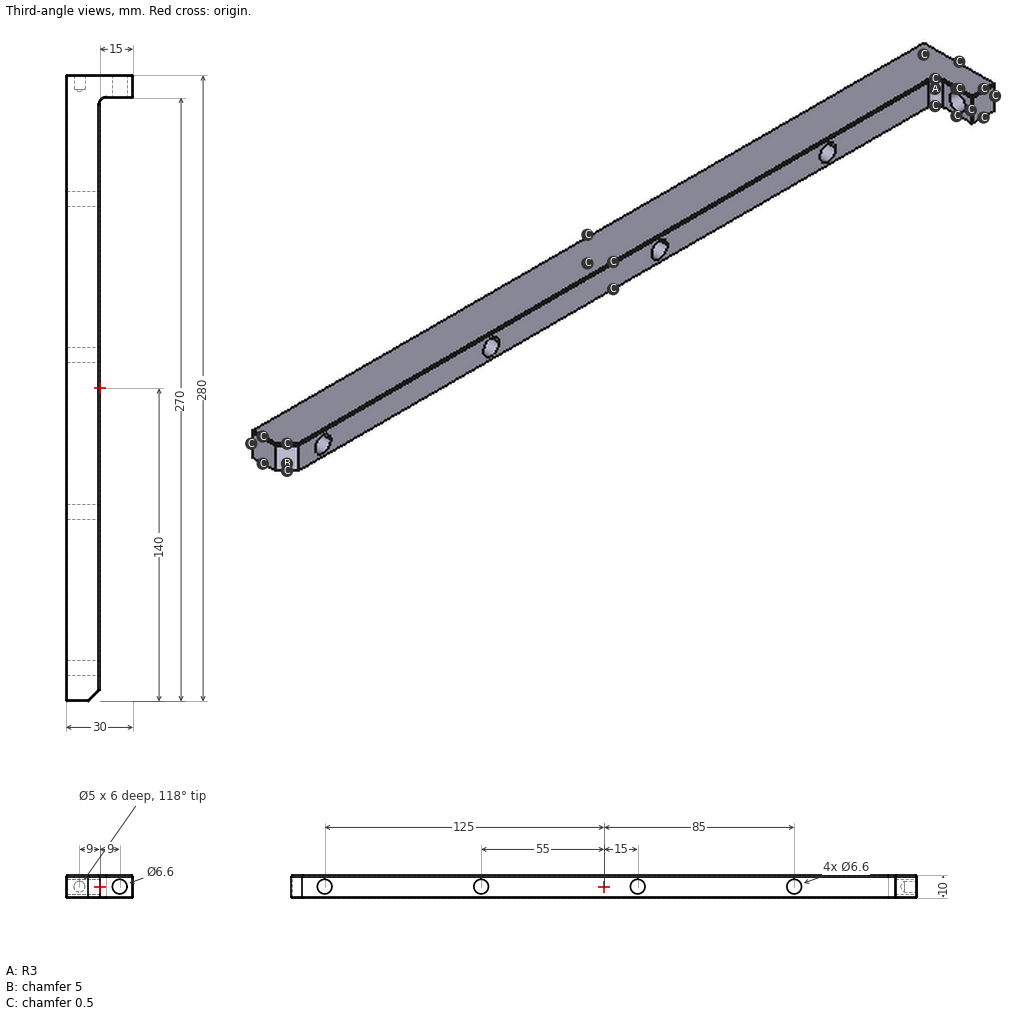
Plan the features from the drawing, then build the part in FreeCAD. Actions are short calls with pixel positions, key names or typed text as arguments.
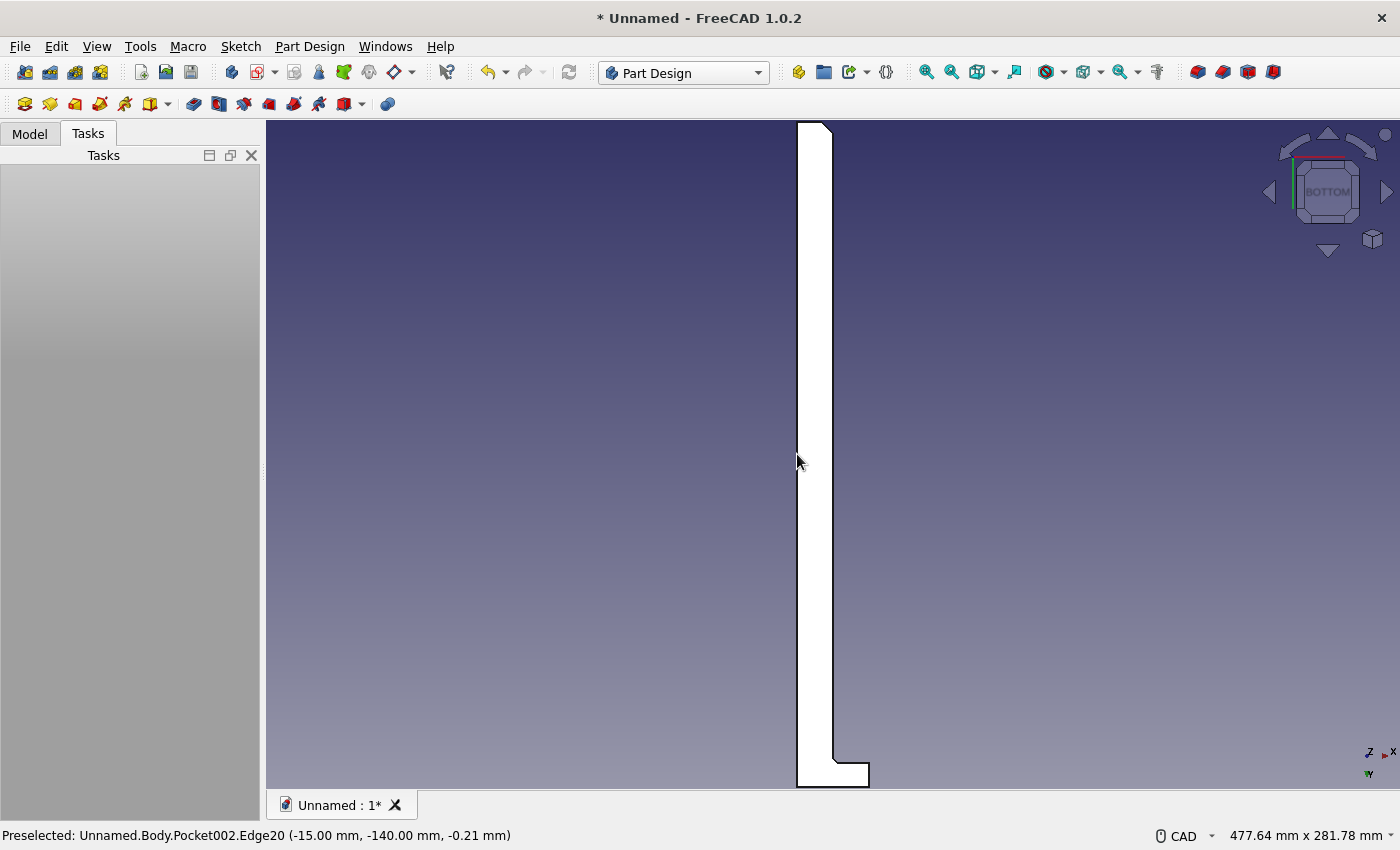
click(813, 738, ctrl)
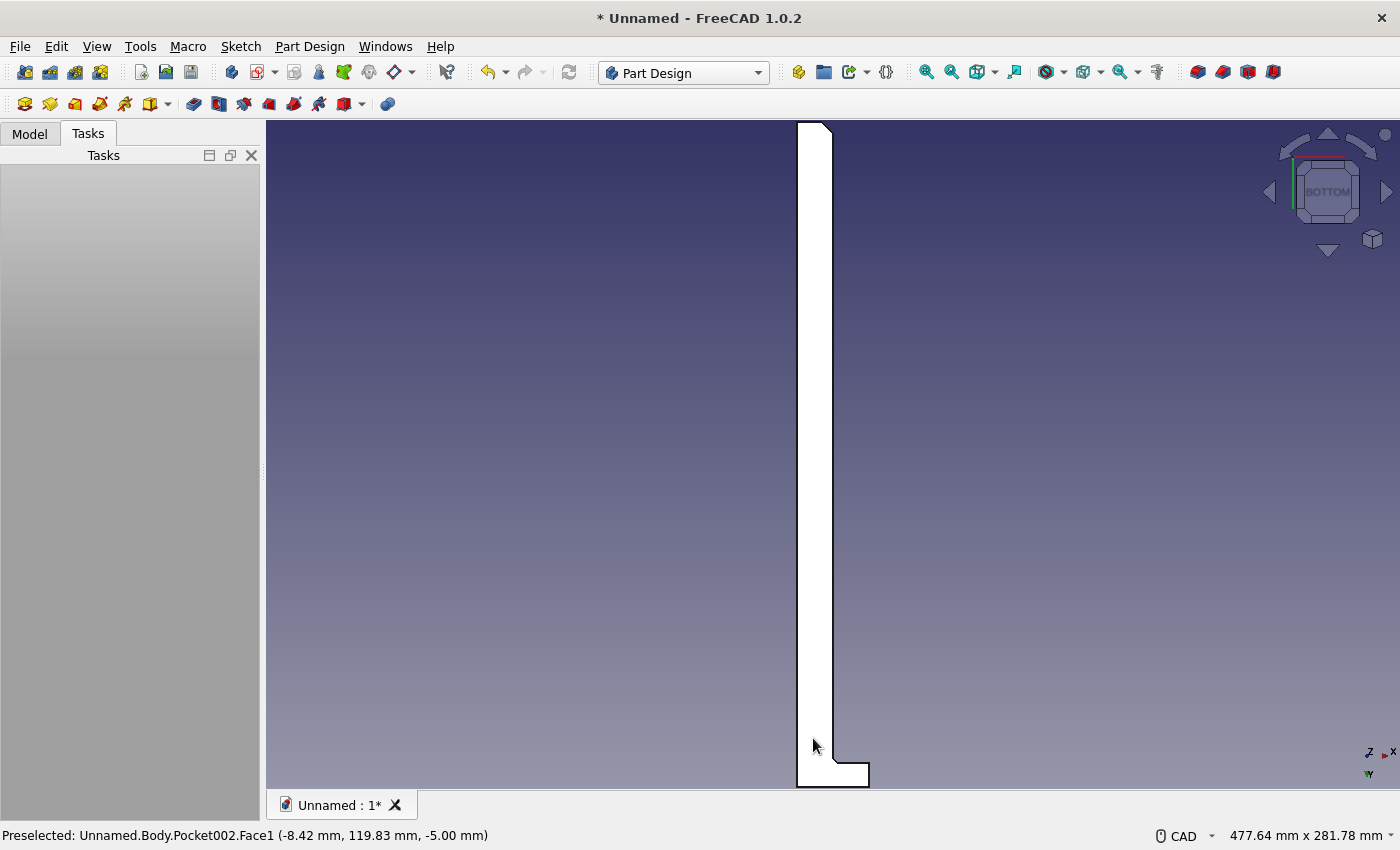
key(4)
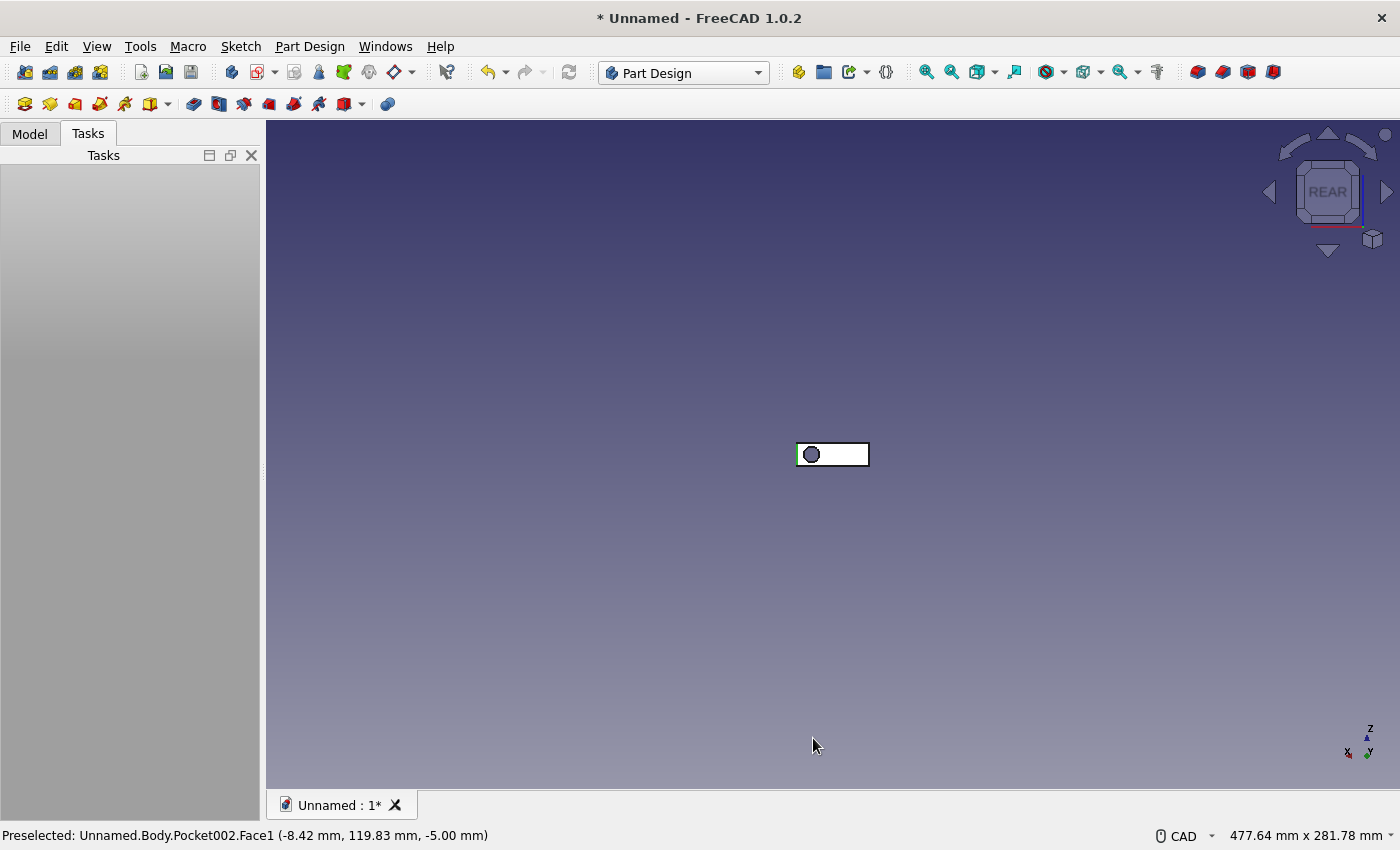
key(v)
key(f)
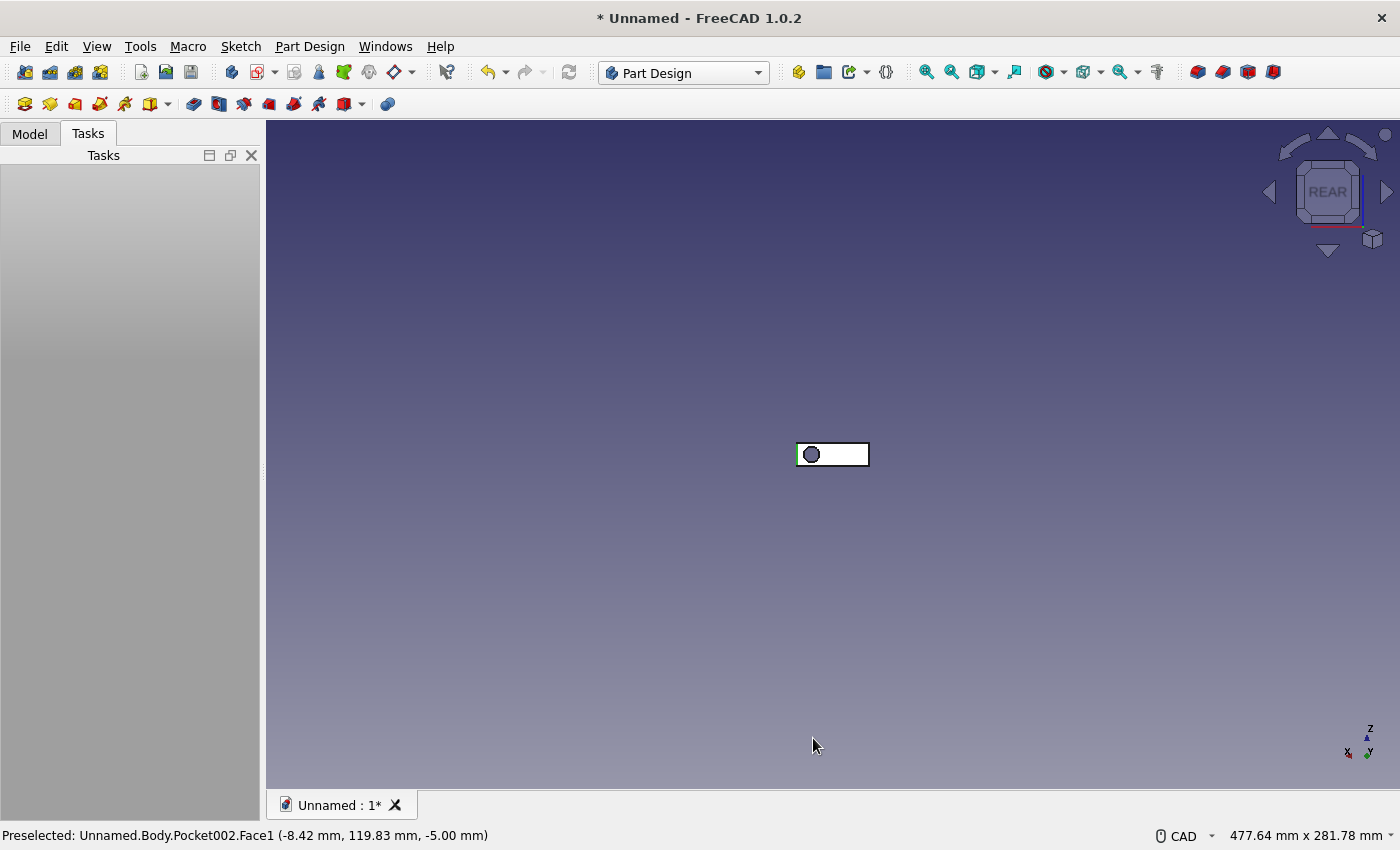
click(869, 454, ctrl)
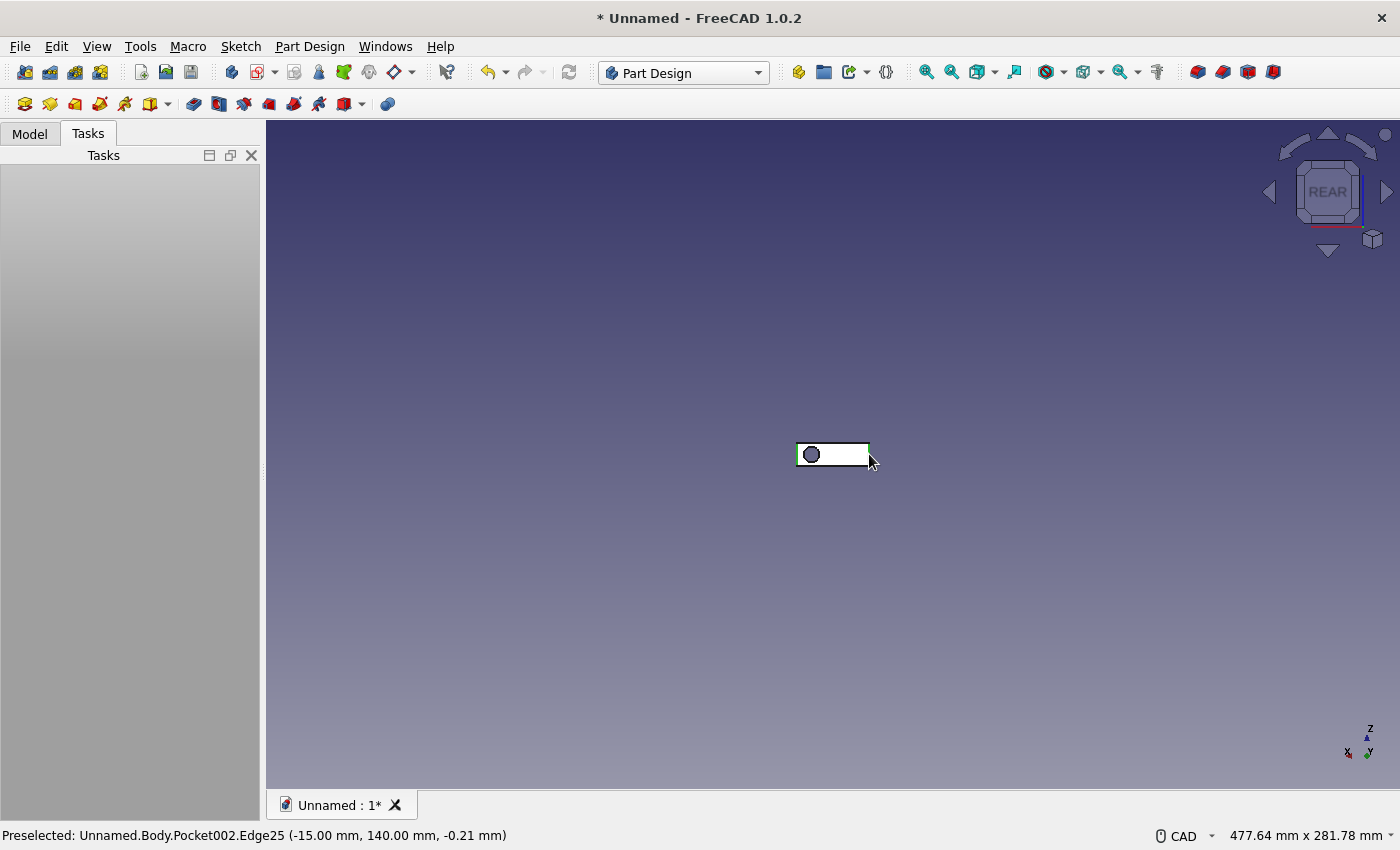
click(1223, 72)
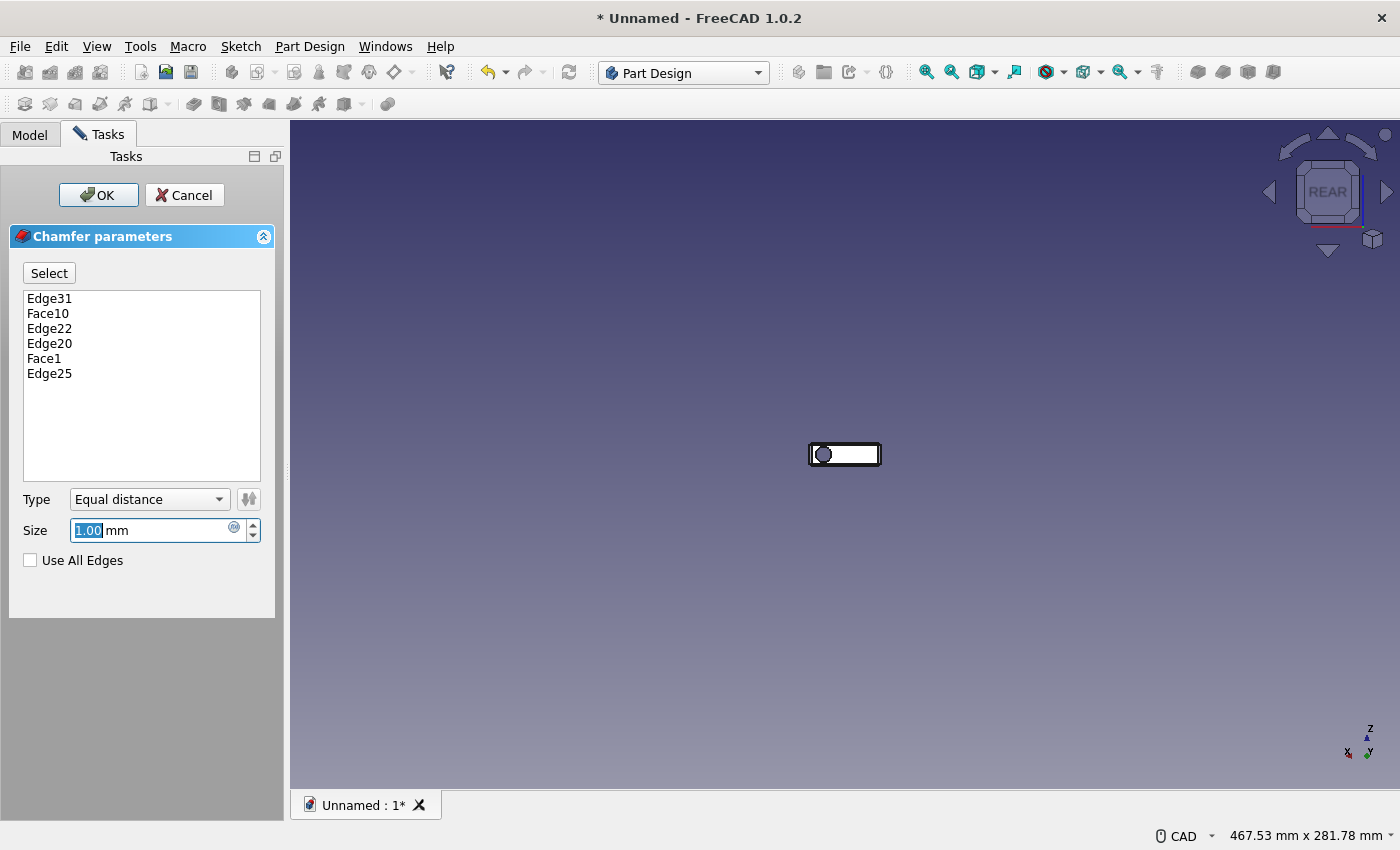
text(0.5)
key(Tab)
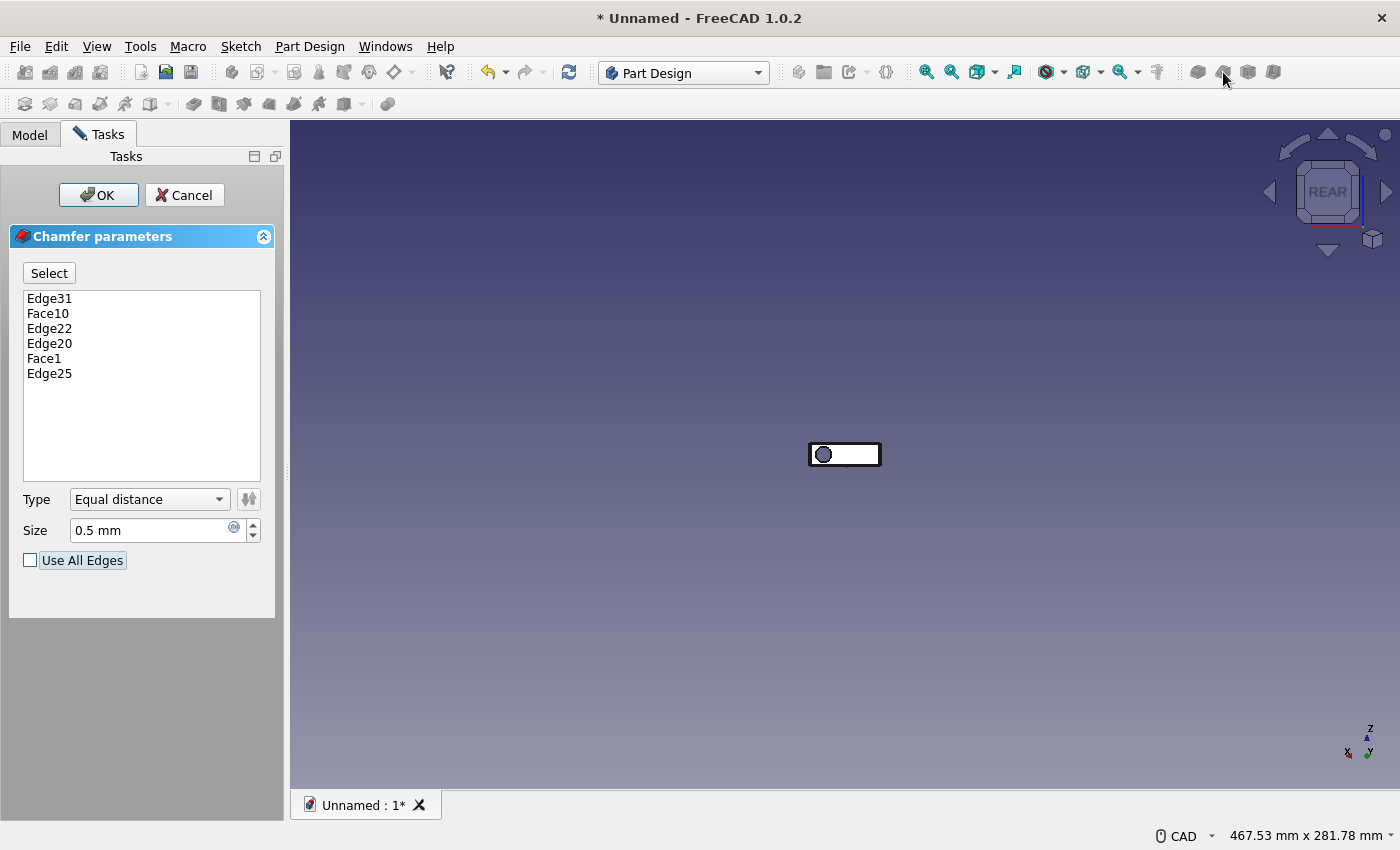
click(99, 195)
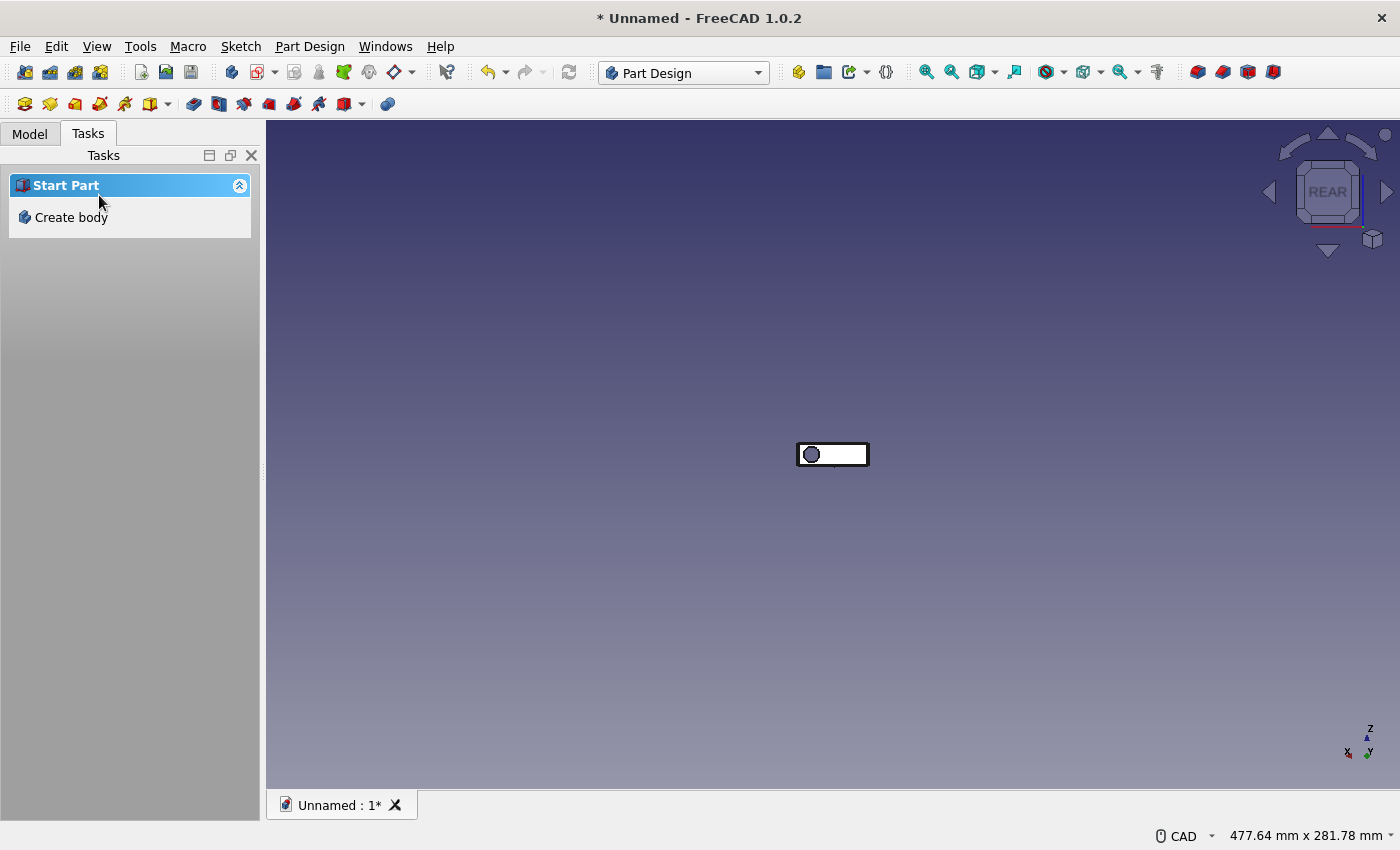
click(927, 72)